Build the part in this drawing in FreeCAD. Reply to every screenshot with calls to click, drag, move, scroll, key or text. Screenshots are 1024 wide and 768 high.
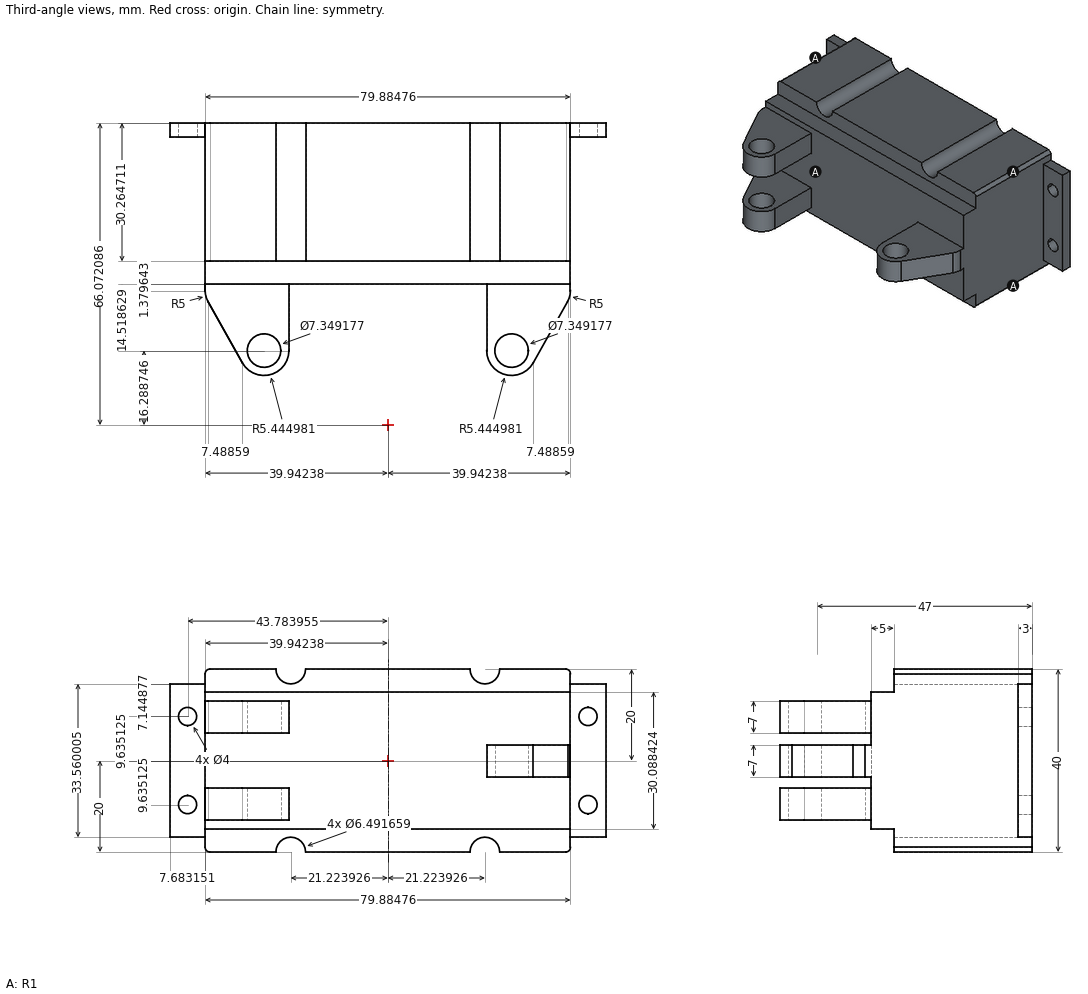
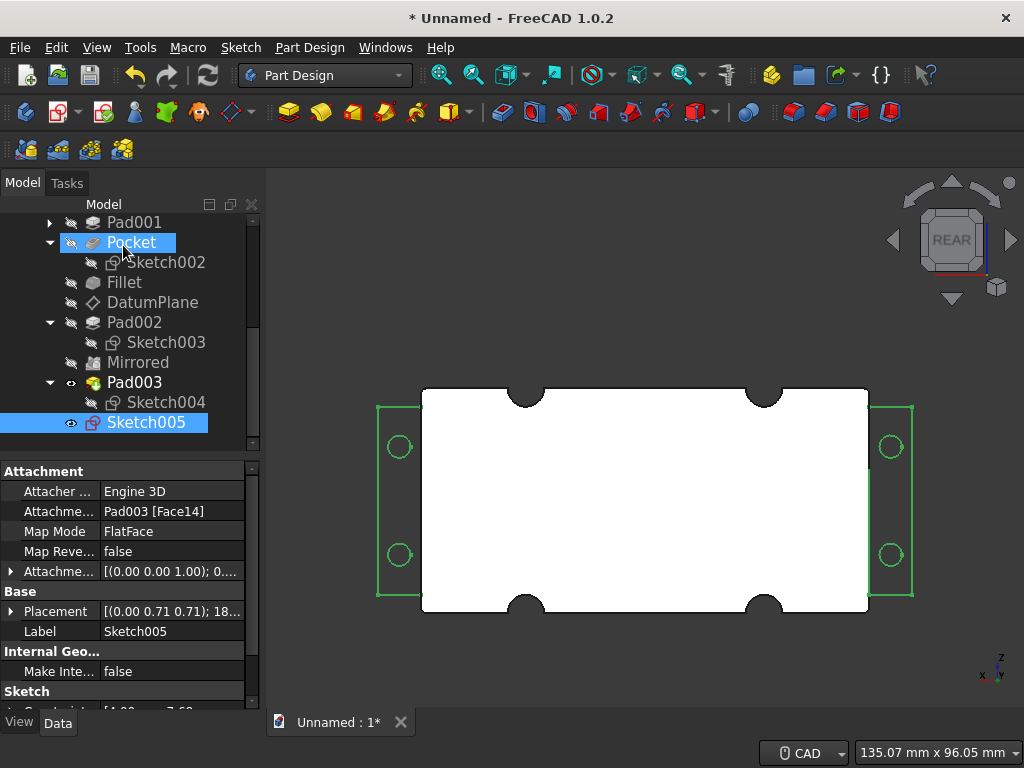
click(290, 112)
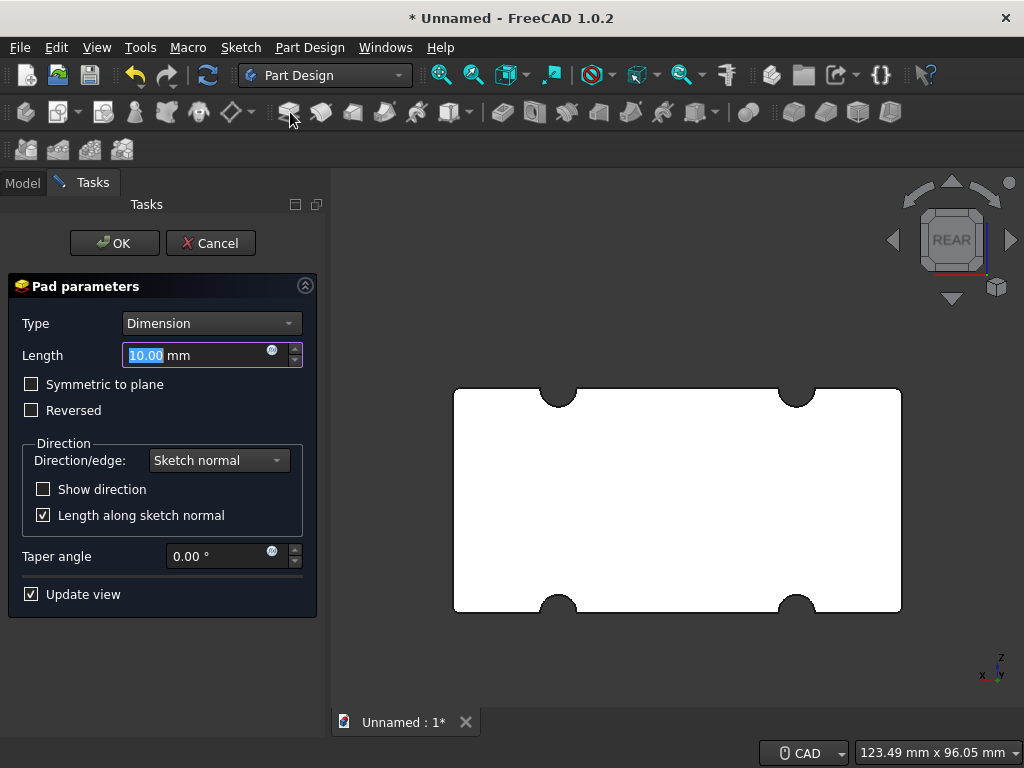
text(3)
key(Tab)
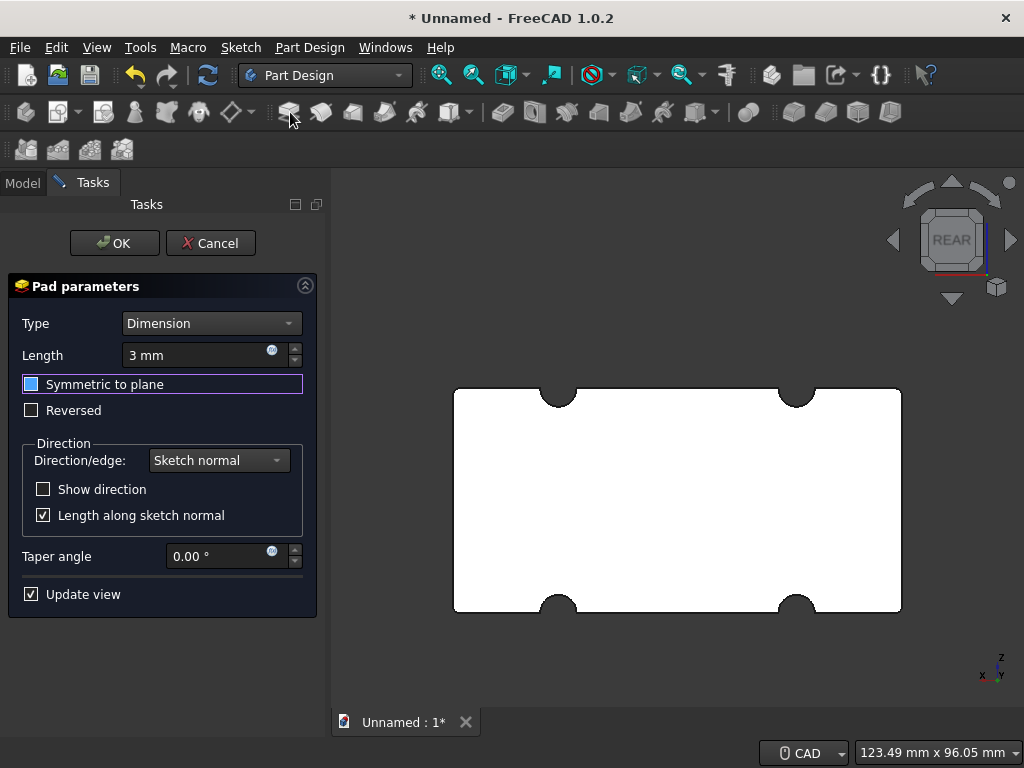
click(30, 410)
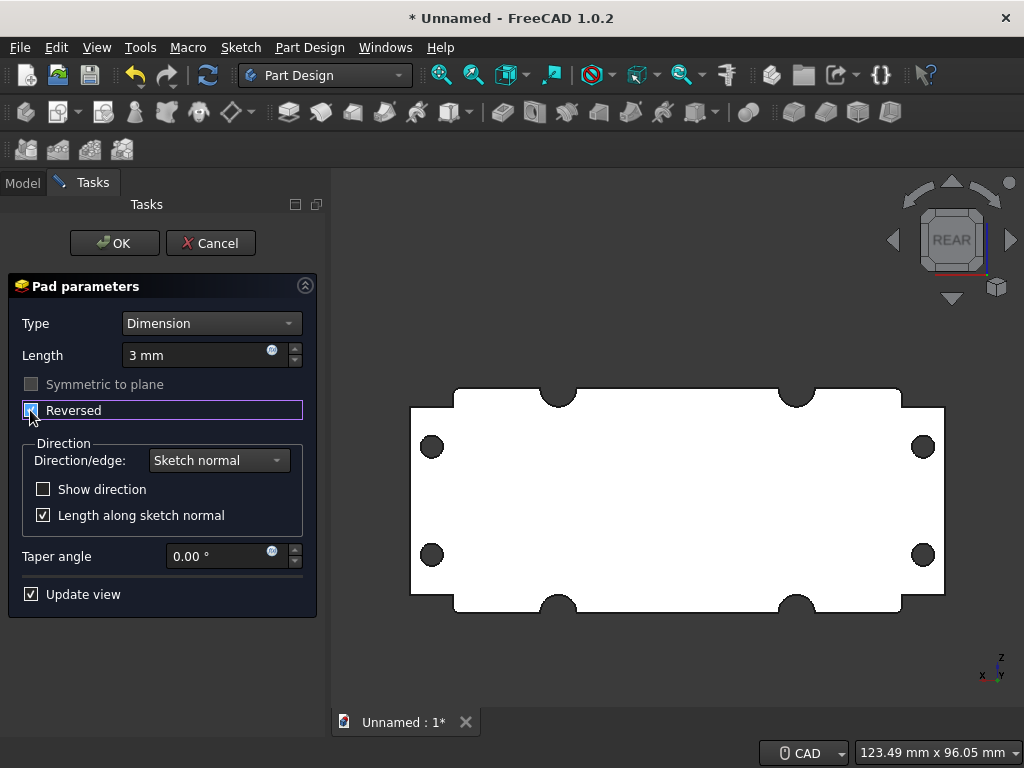
click(115, 243)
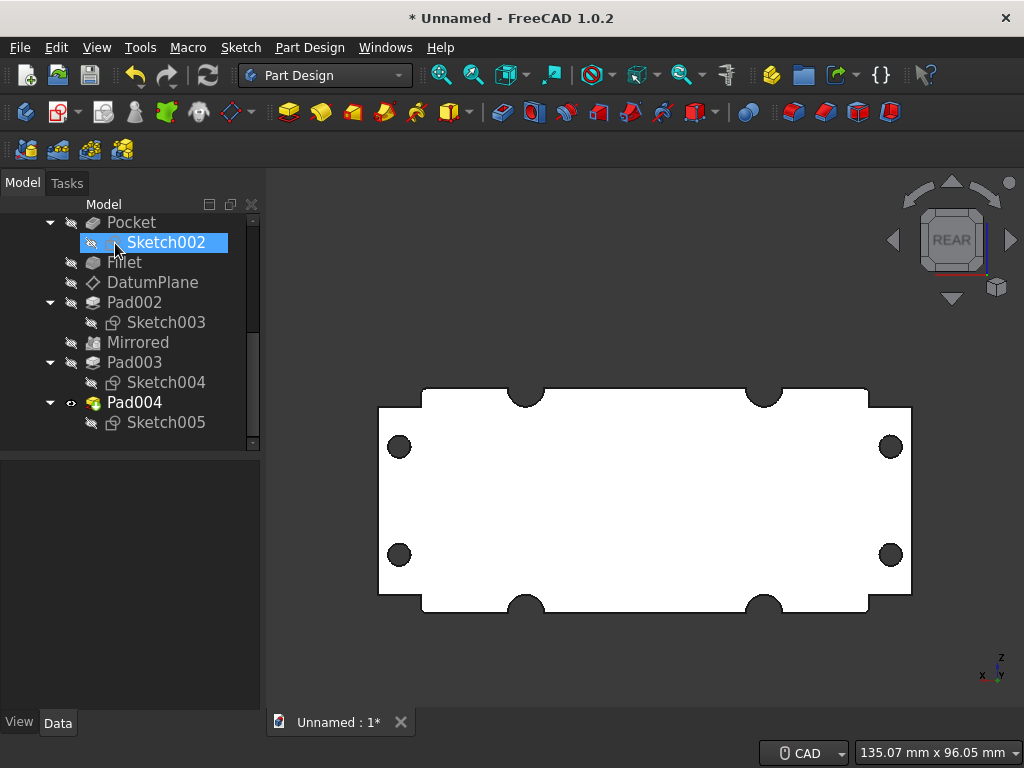
key(0)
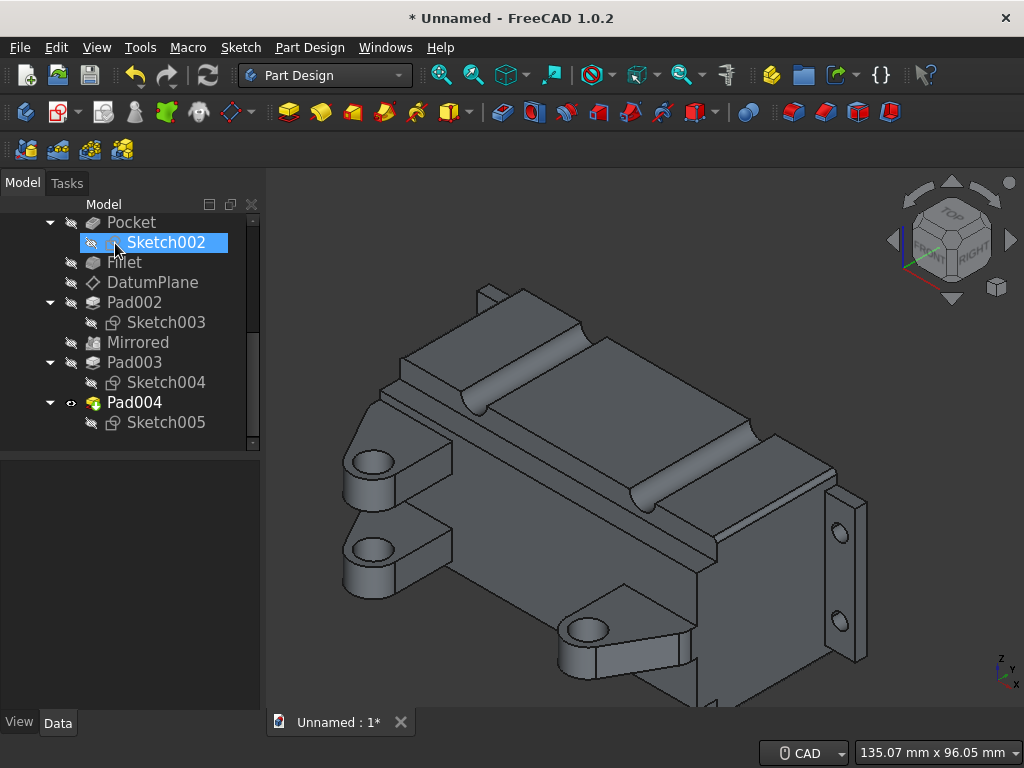
key(v)
key(f)